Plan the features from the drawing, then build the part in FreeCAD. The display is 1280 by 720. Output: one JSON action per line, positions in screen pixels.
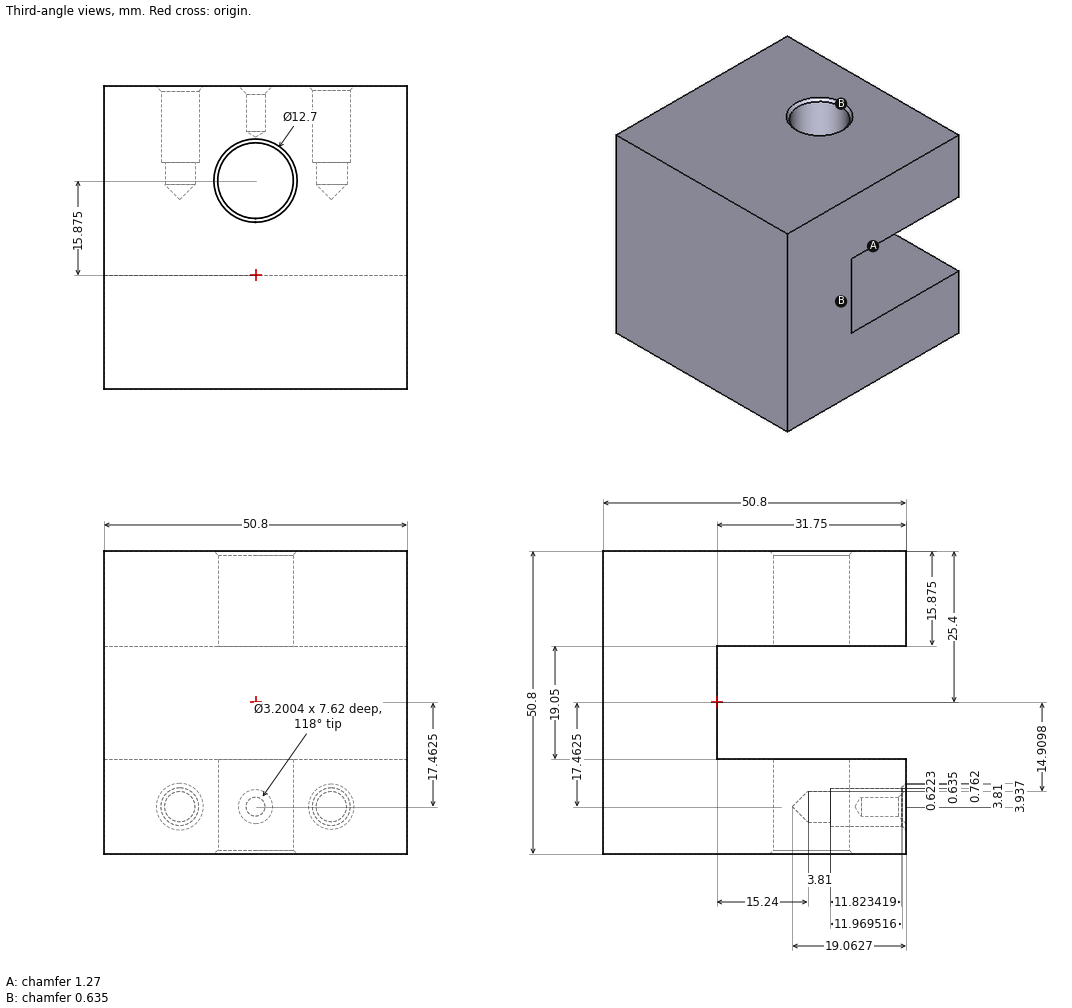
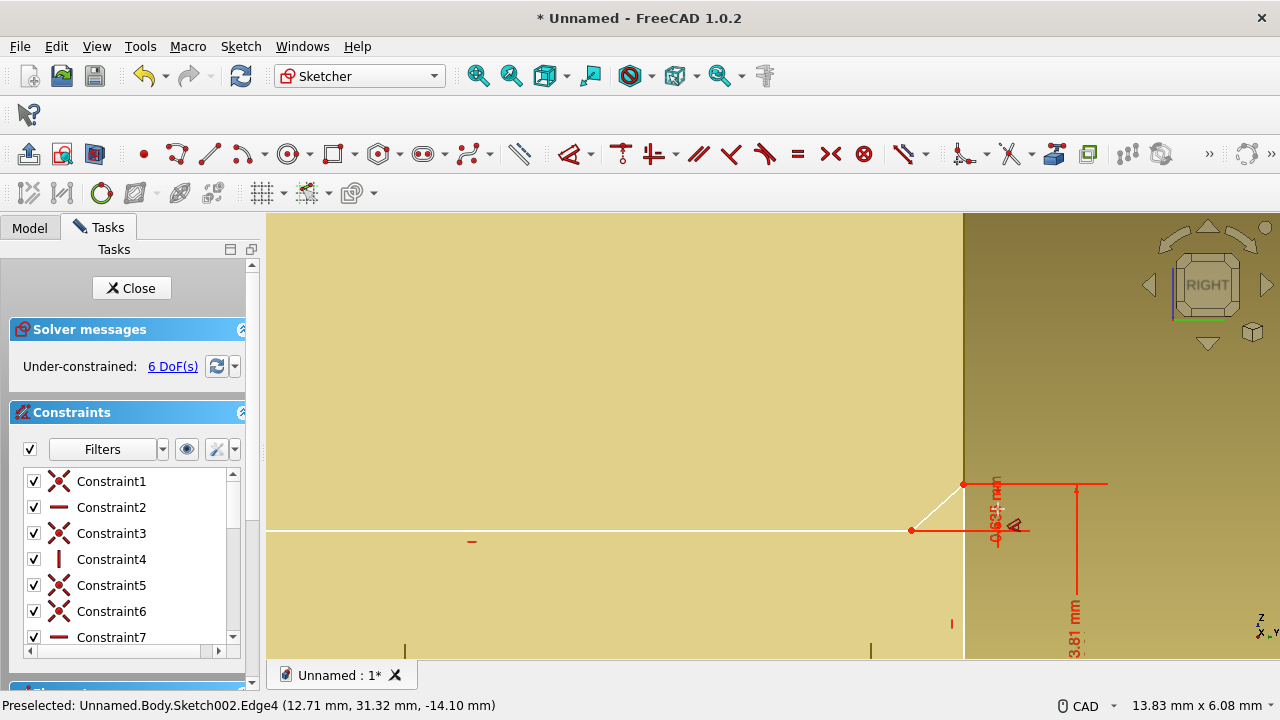
{"action": "scroll", "coordinate": [933, 516], "scroll_direction": "down", "scroll_amount": 8}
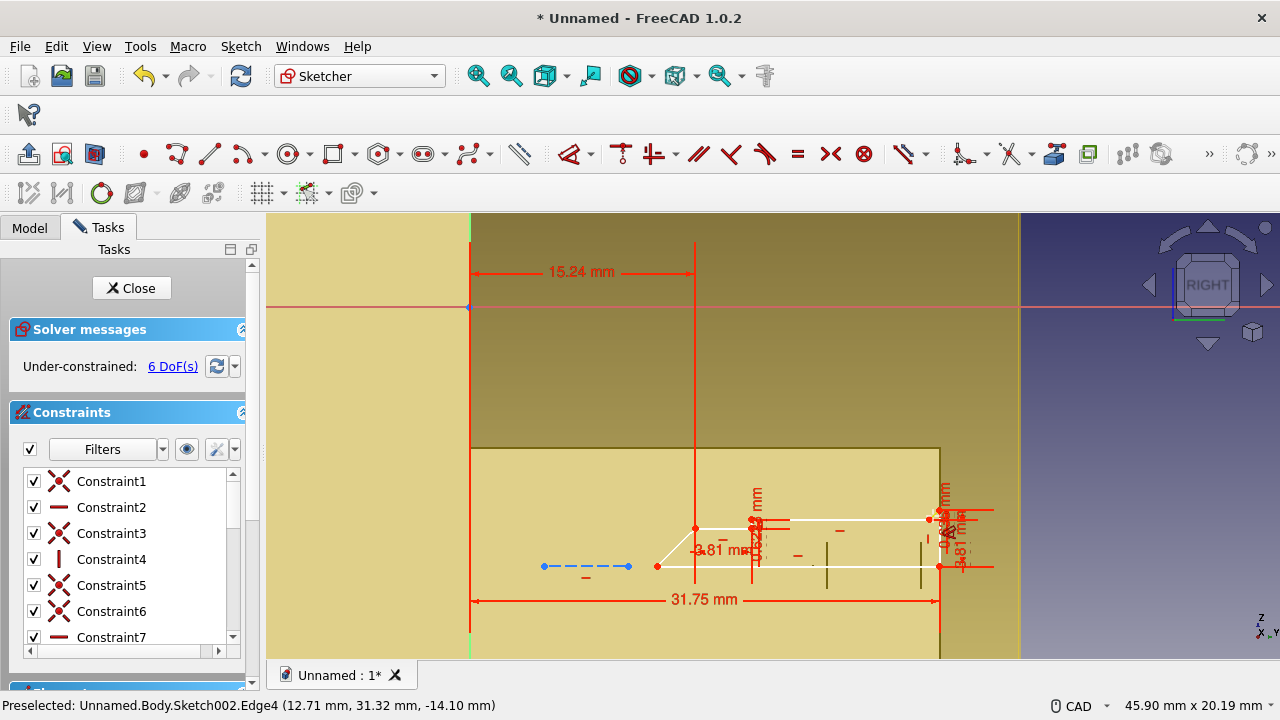
{"action": "left_click", "coordinate": [742, 567]}
{"action": "left_click", "coordinate": [798, 601]}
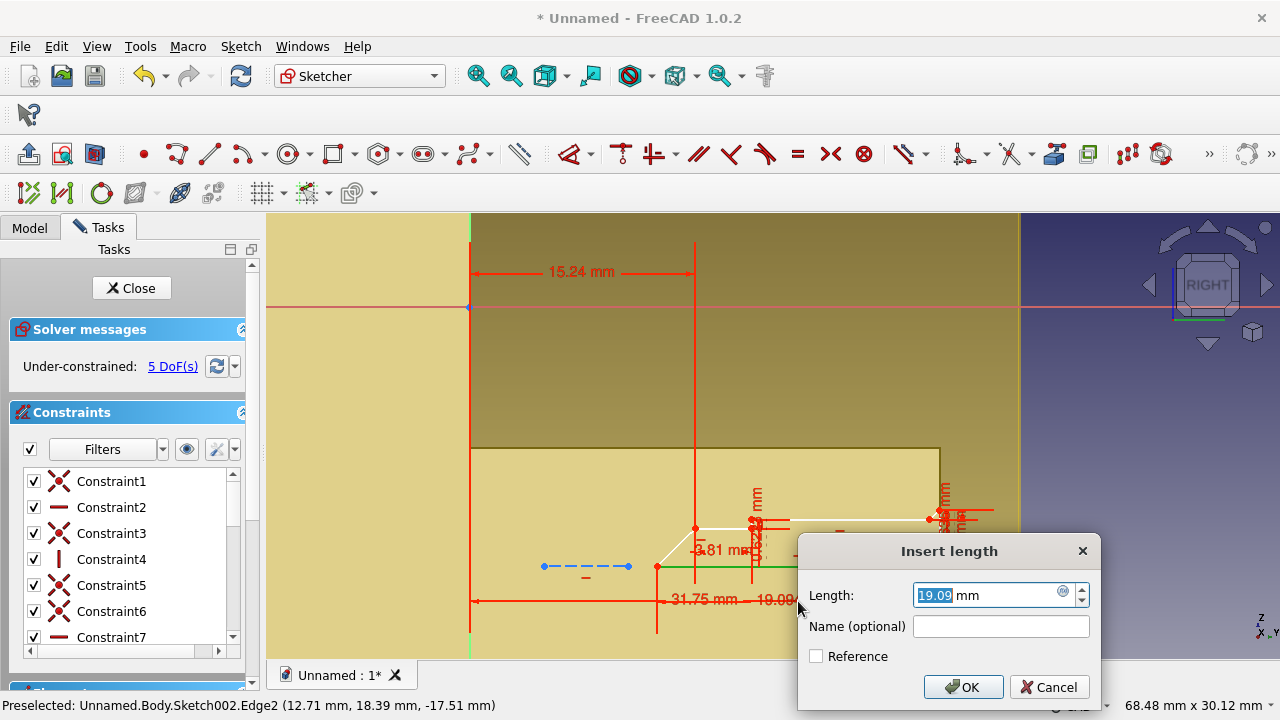
{"action": "type", "text": "19.0627"}
{"action": "key", "text": "Return"}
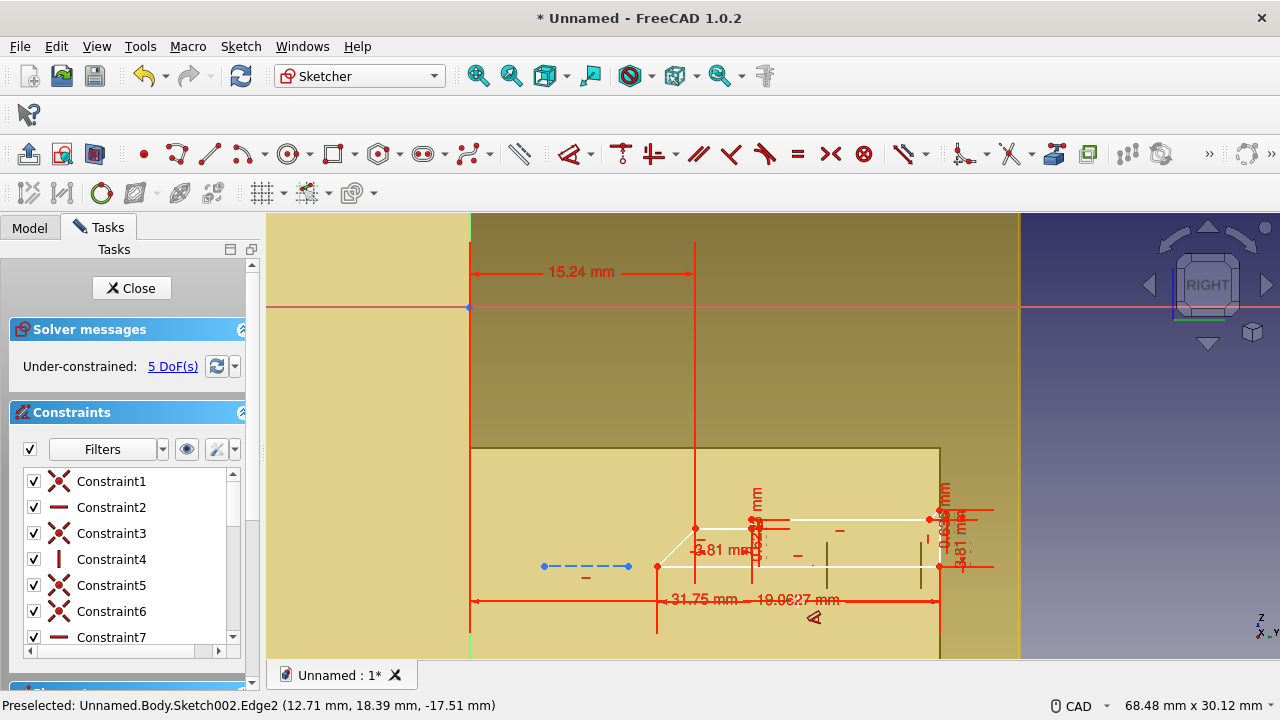
{"action": "left_click", "coordinate": [695, 529]}
{"action": "left_click", "coordinate": [436, 418]}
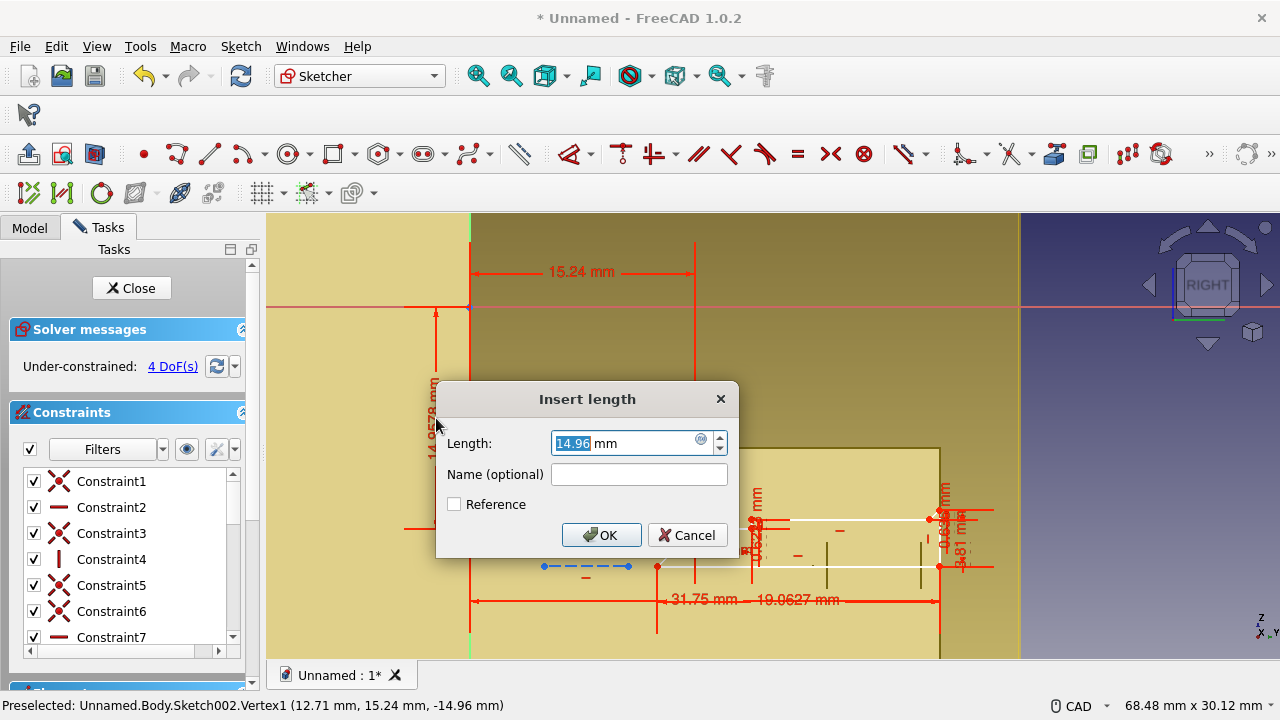
{"action": "type", "text": "14.9098"}
{"action": "key", "text": "Return"}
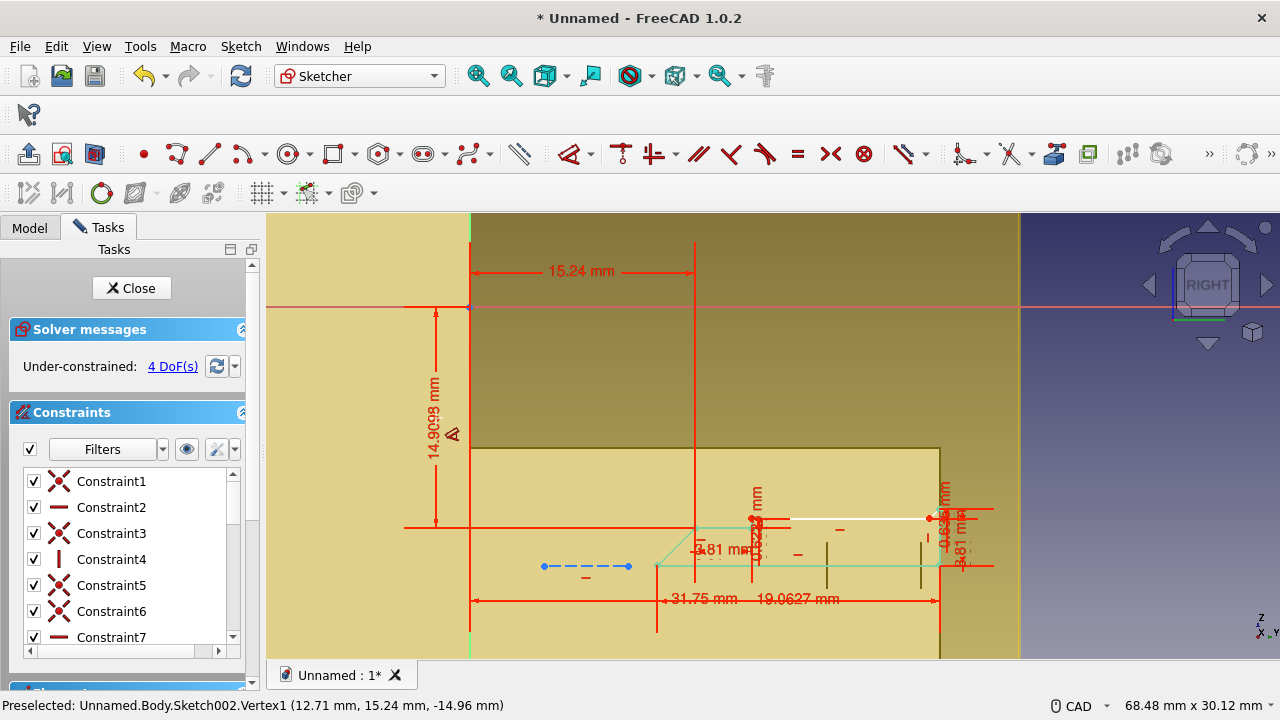
{"action": "left_click", "coordinate": [629, 566]}
{"action": "left_click", "coordinate": [436, 377]}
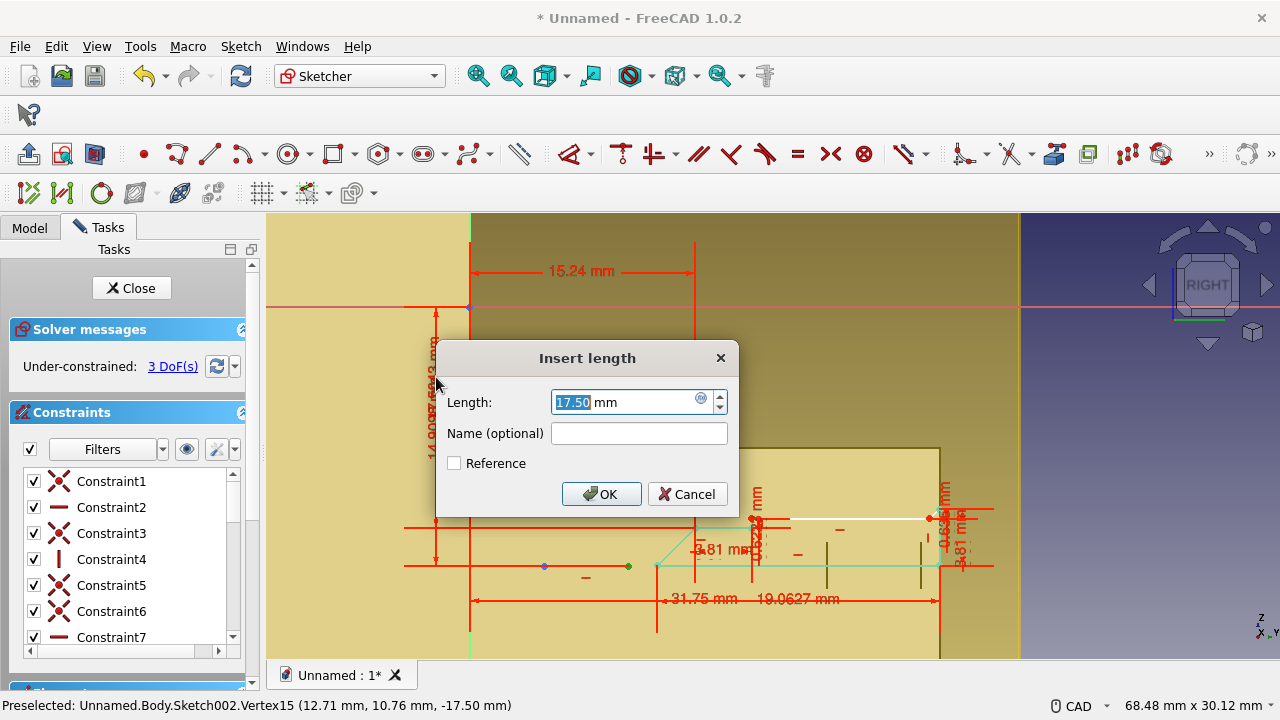
{"action": "type", "text": "17.4625"}
{"action": "key", "text": "Return"}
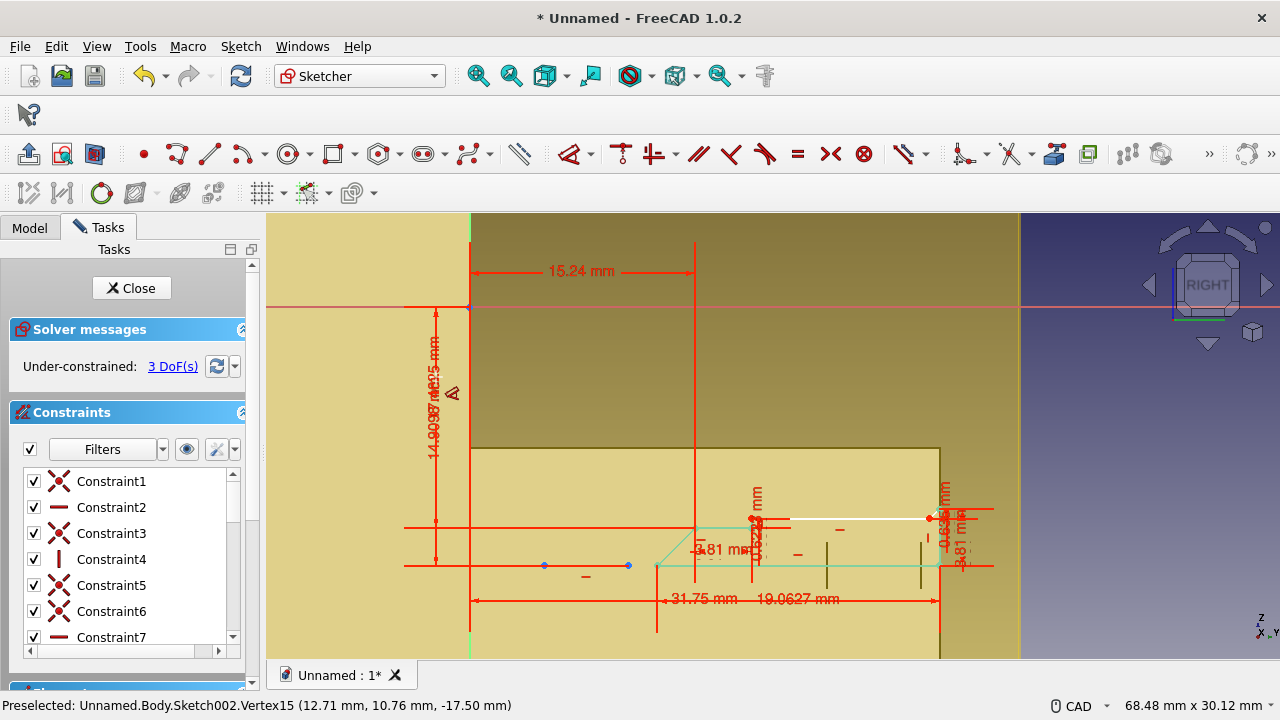
{"action": "left_click", "coordinate": [876, 519]}
{"action": "left_click", "coordinate": [840, 553]}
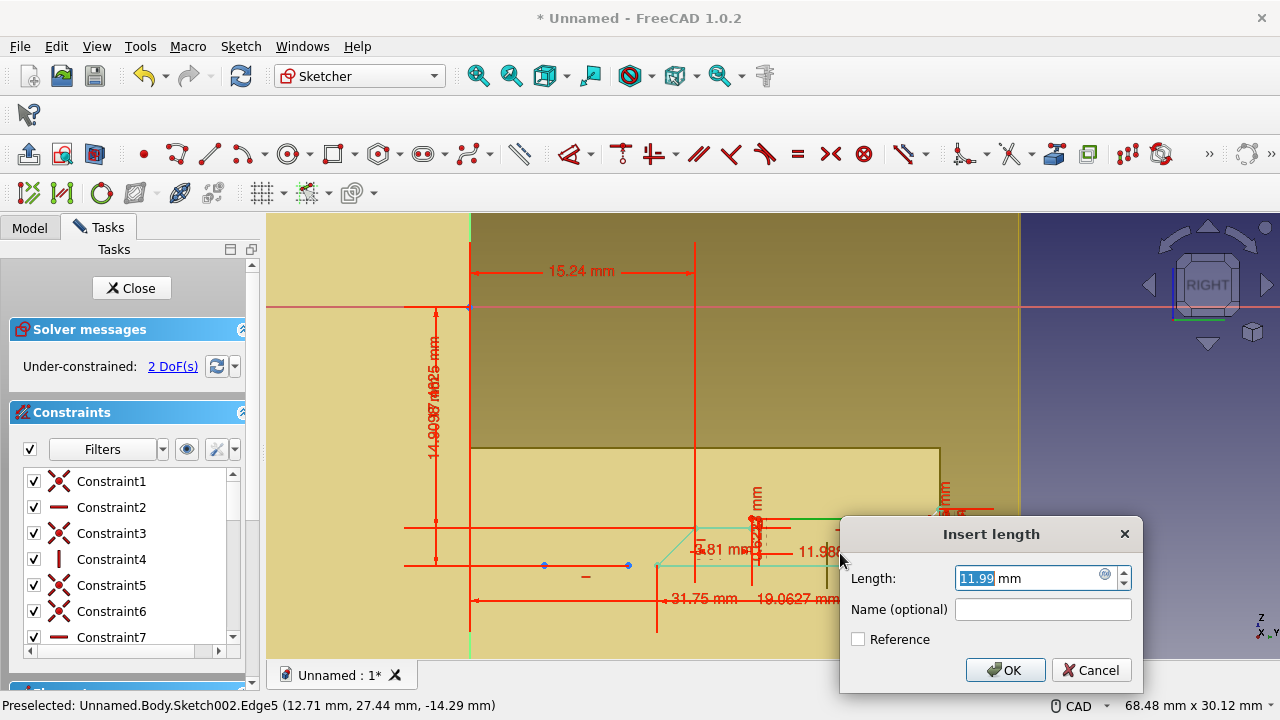
{"action": "type", "text": "11.969516"}
{"action": "key", "text": "Return"}
{"action": "key", "text": "Escape"}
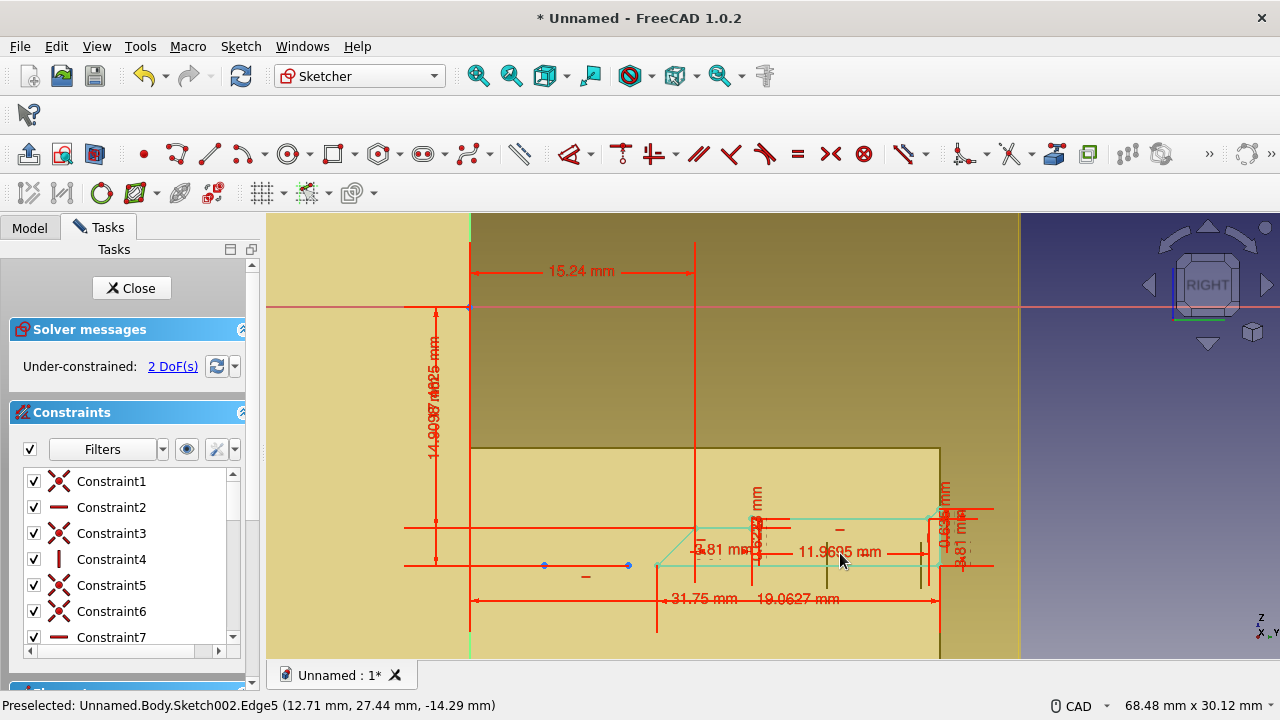
{"action": "left_click", "coordinate": [132, 288]}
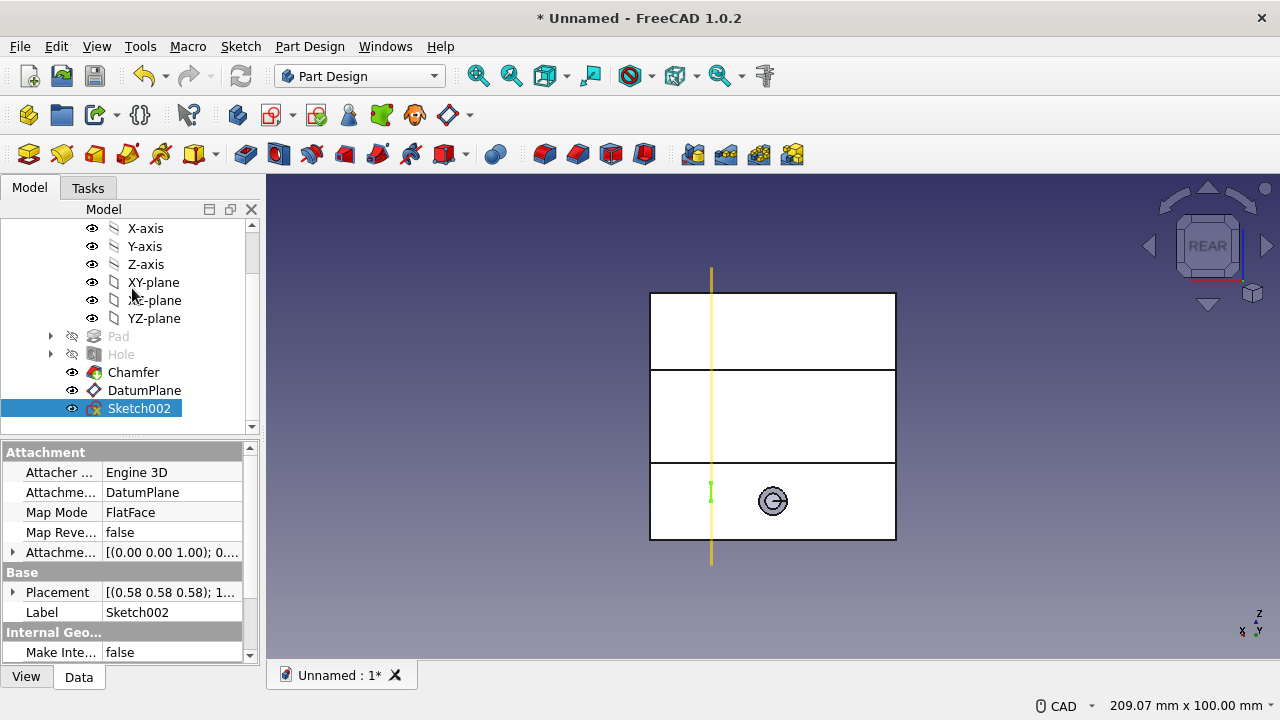
{"action": "left_click", "coordinate": [312, 154]}